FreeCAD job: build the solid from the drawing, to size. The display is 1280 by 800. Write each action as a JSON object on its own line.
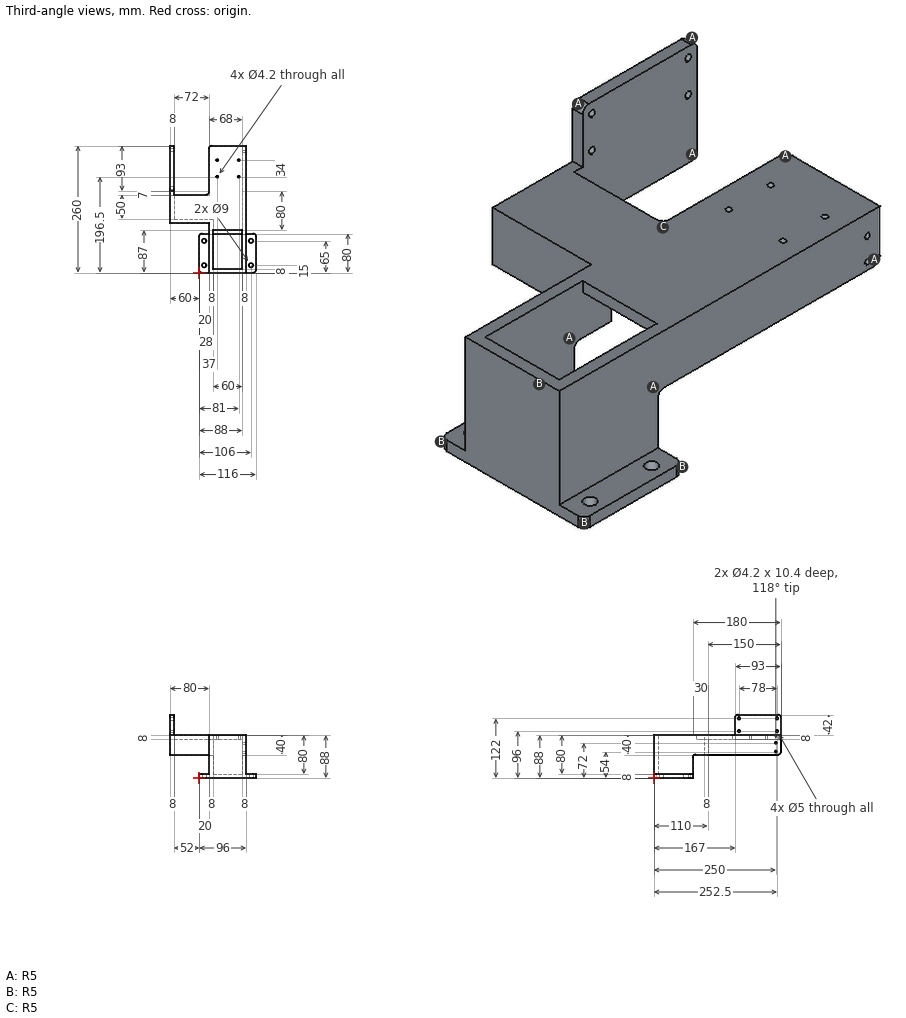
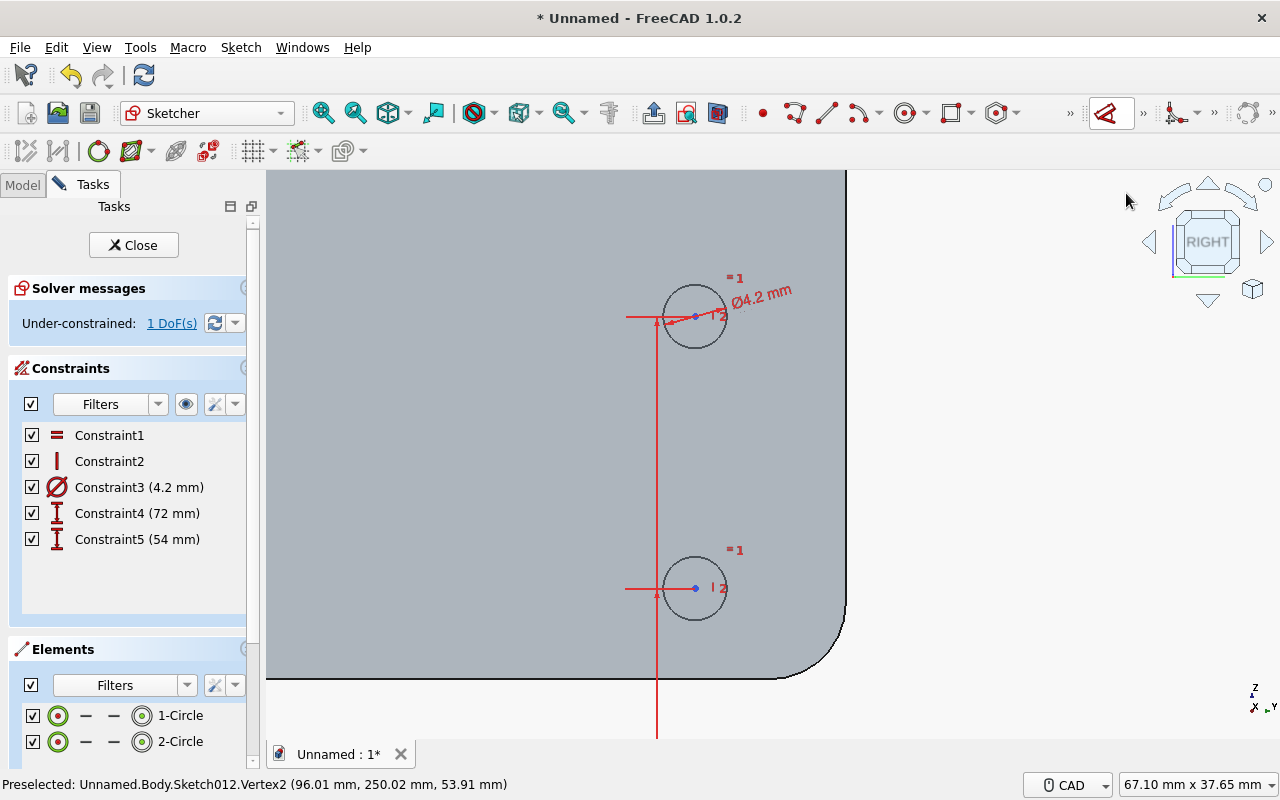
{"action": "left_click", "coordinate": [695, 317]}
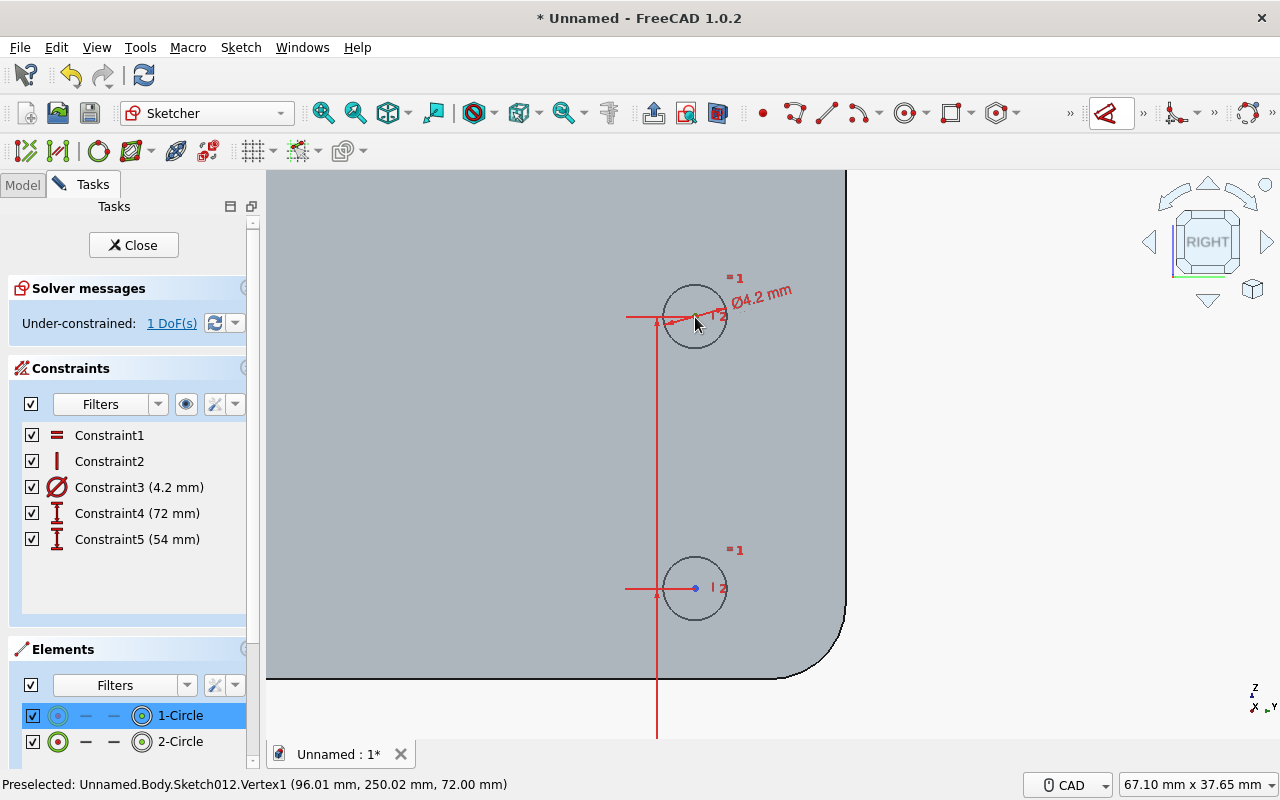
{"action": "left_click", "coordinate": [1128, 114]}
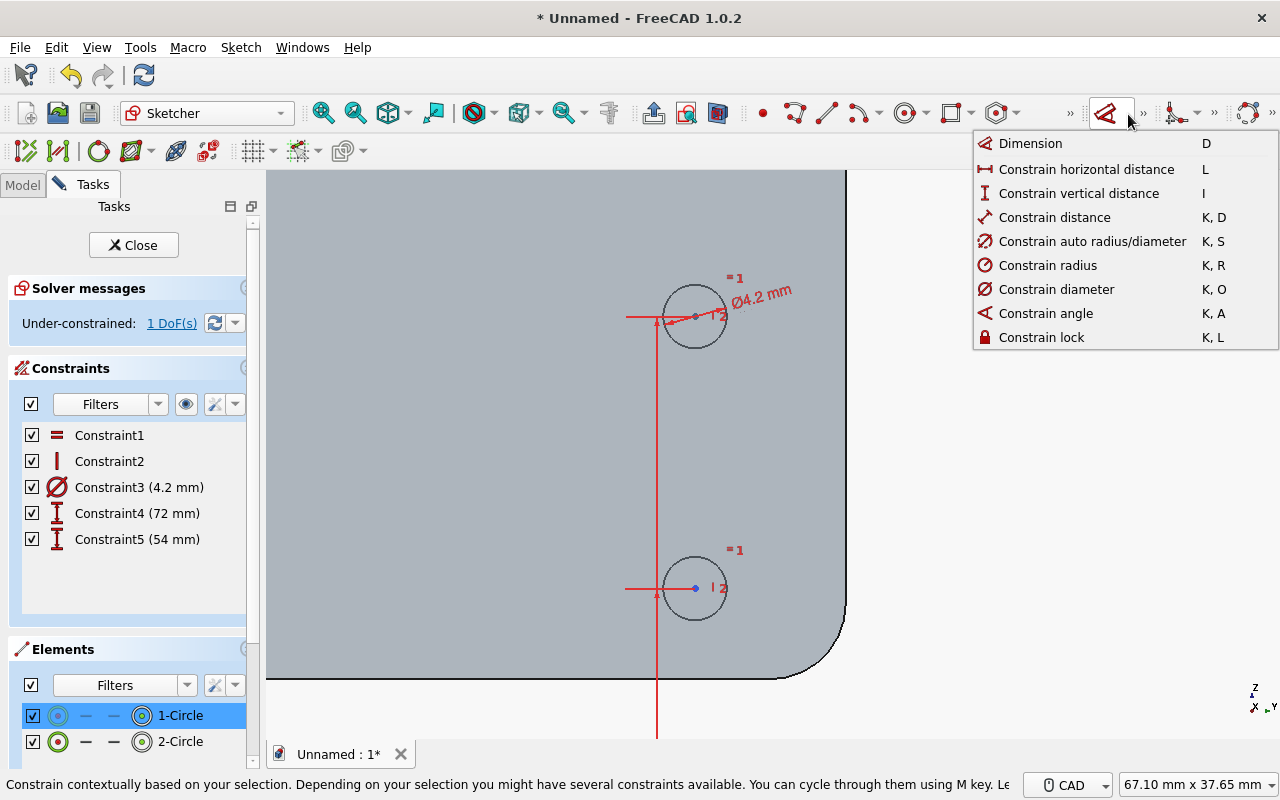
{"action": "left_click", "coordinate": [1126, 169]}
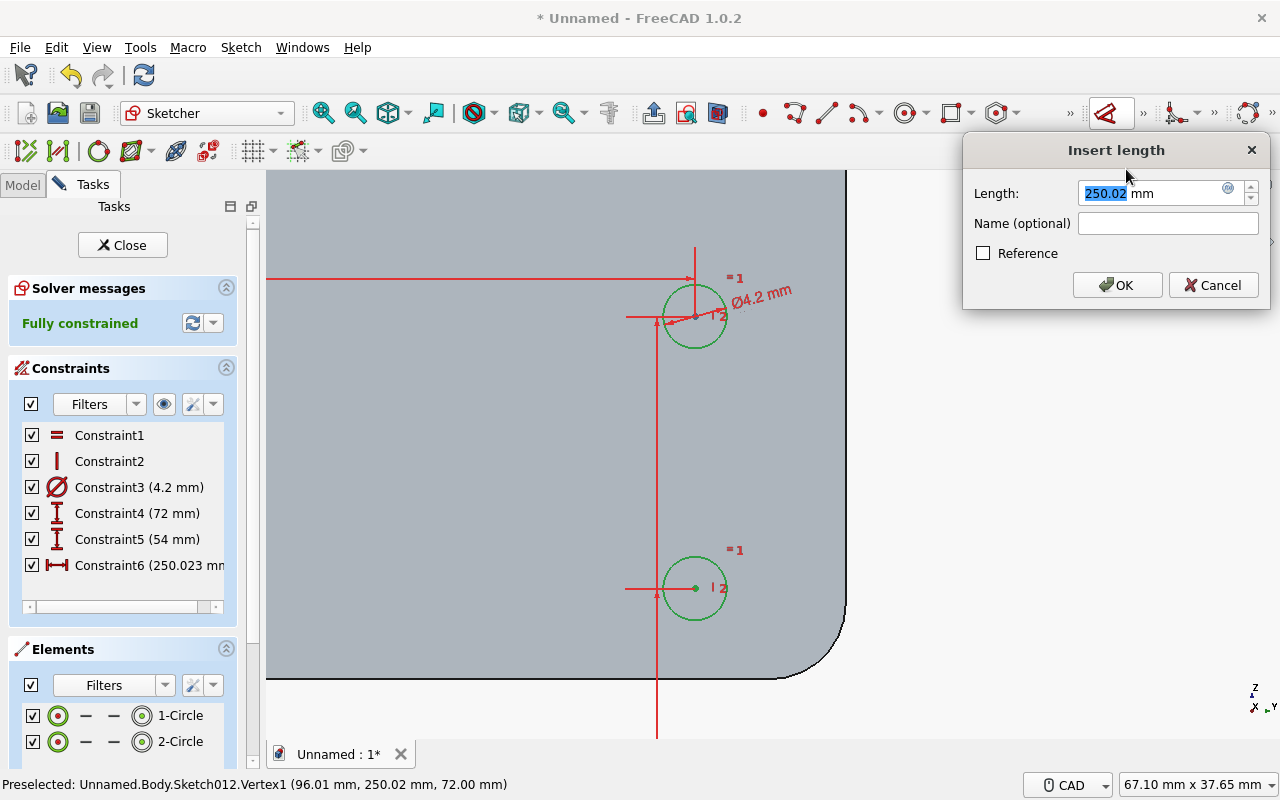
{"action": "type", "text": "250"}
{"action": "key", "text": "Return"}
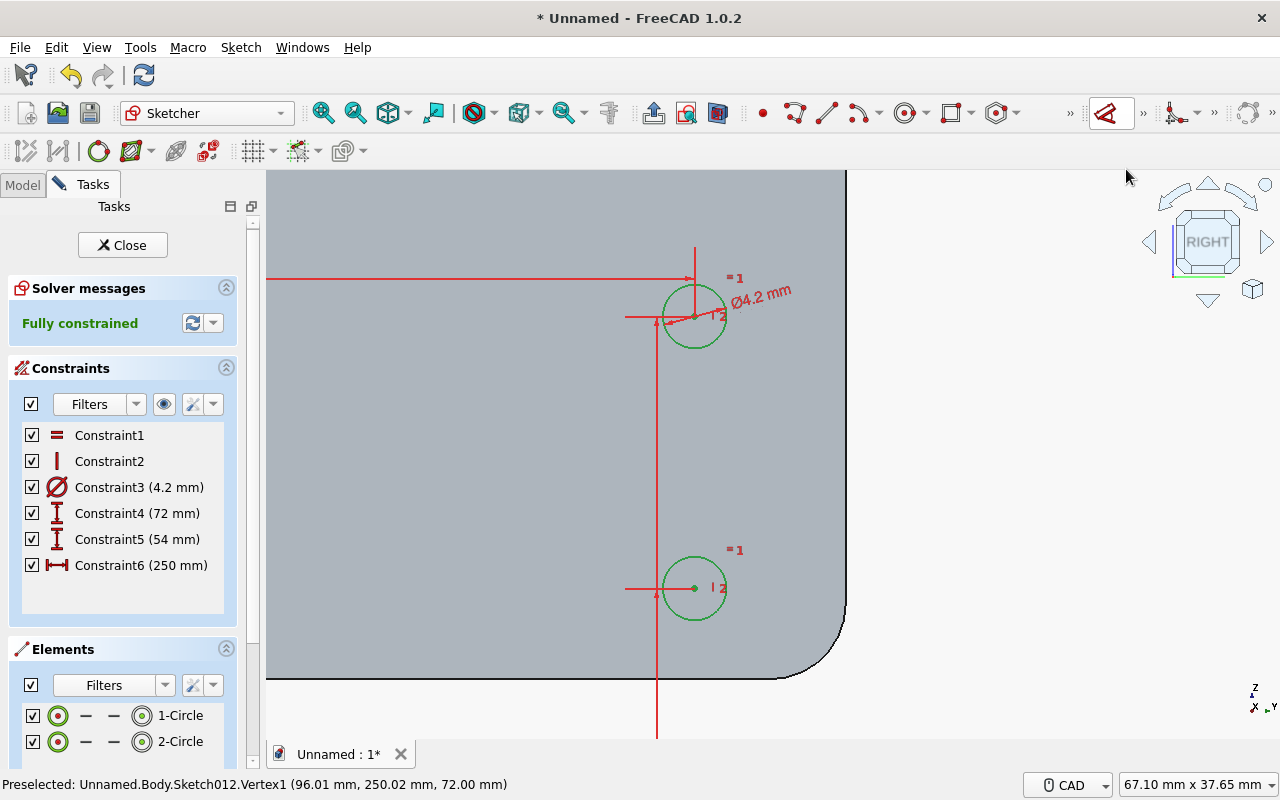
{"action": "left_click", "coordinate": [123, 245]}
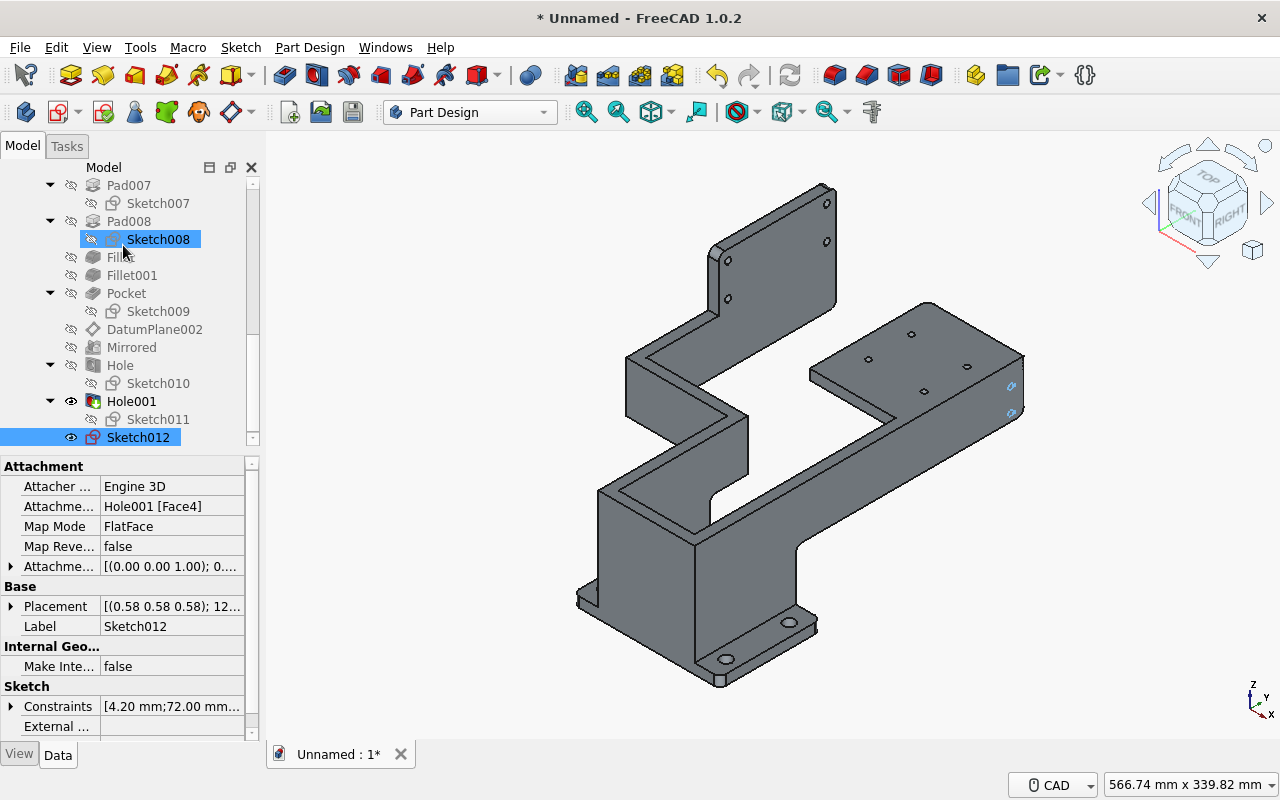
{"action": "left_click", "coordinate": [318, 76]}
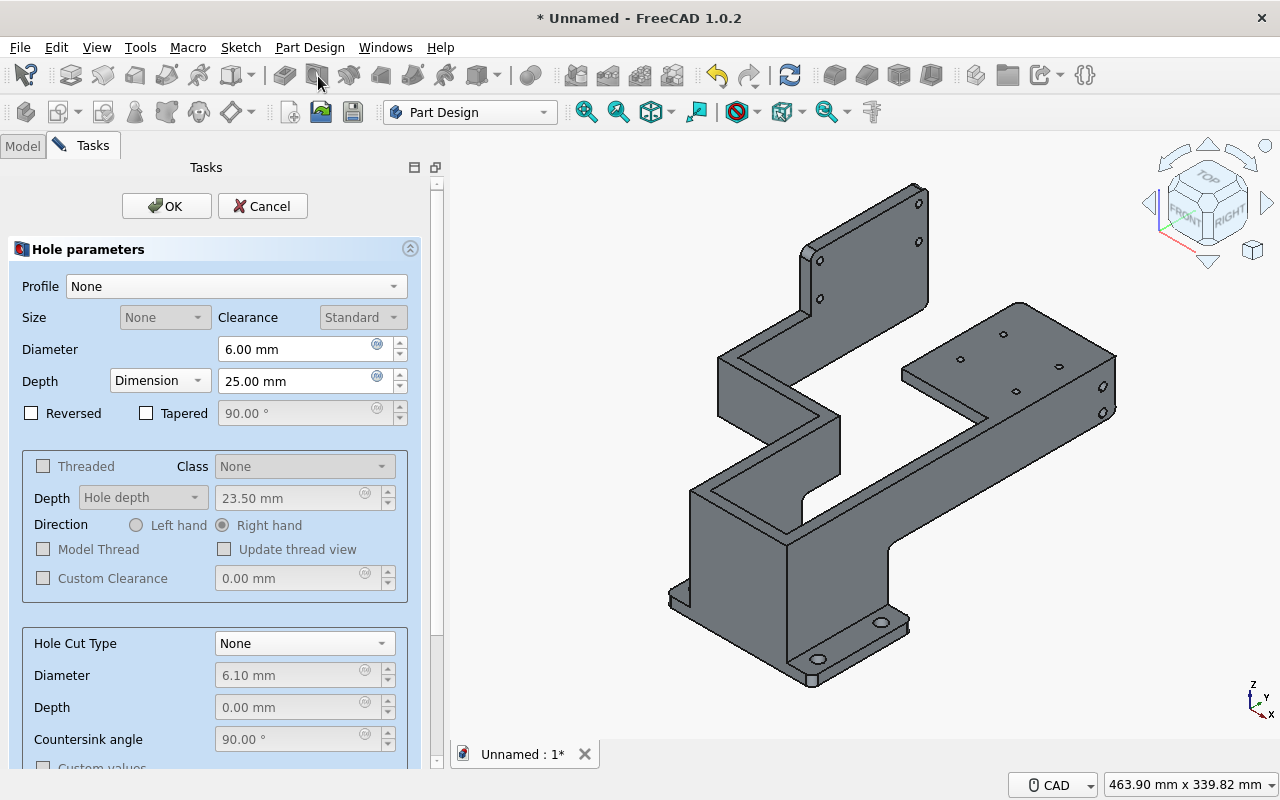
{"action": "triple_click", "coordinate": [305, 349]}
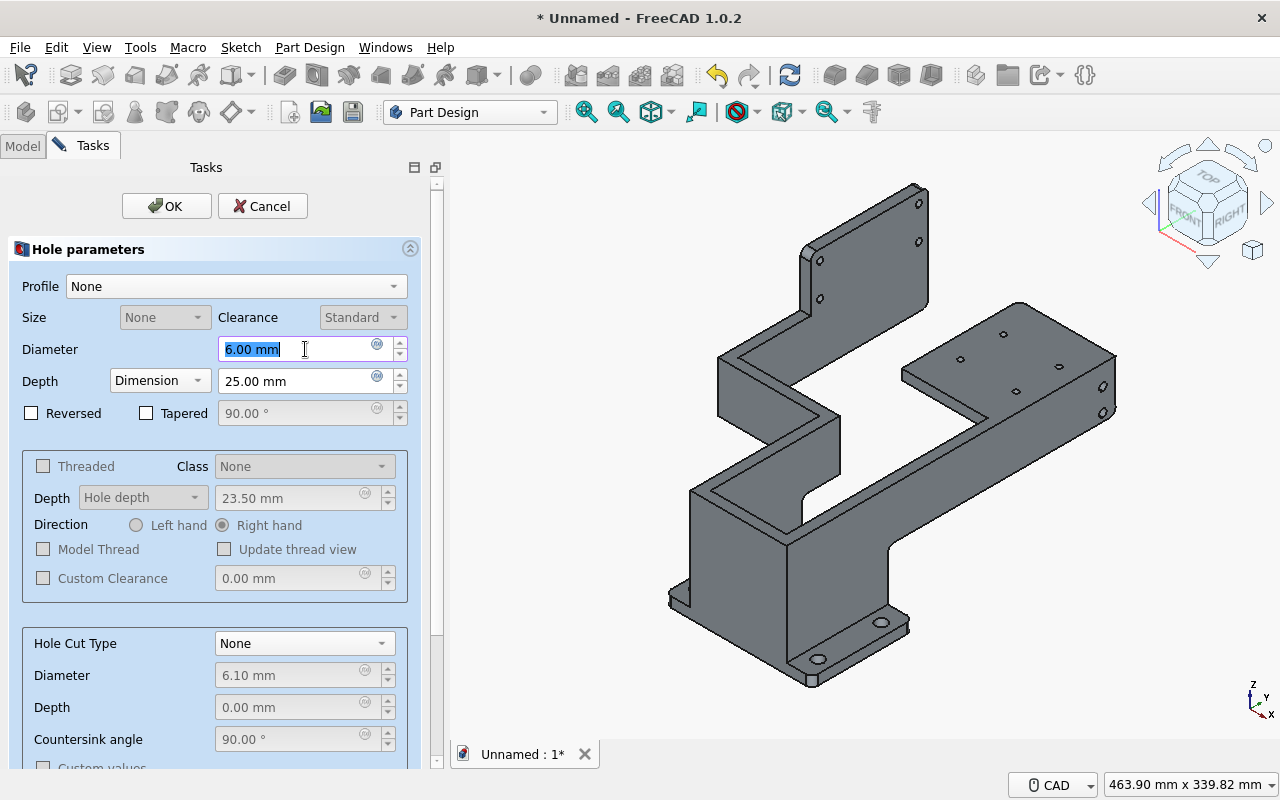
{"action": "type", "text": "4.2"}
{"action": "key", "text": "Tab"}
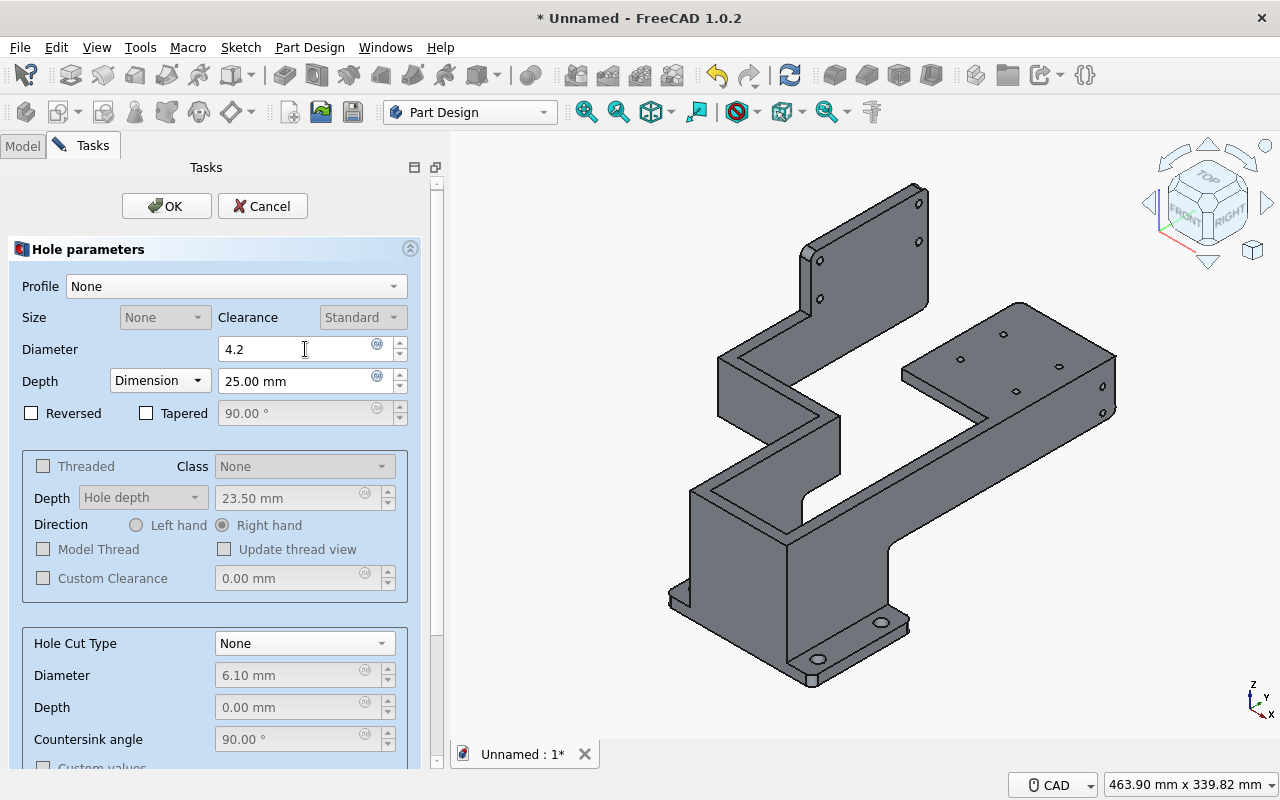
{"action": "triple_click", "coordinate": [305, 381]}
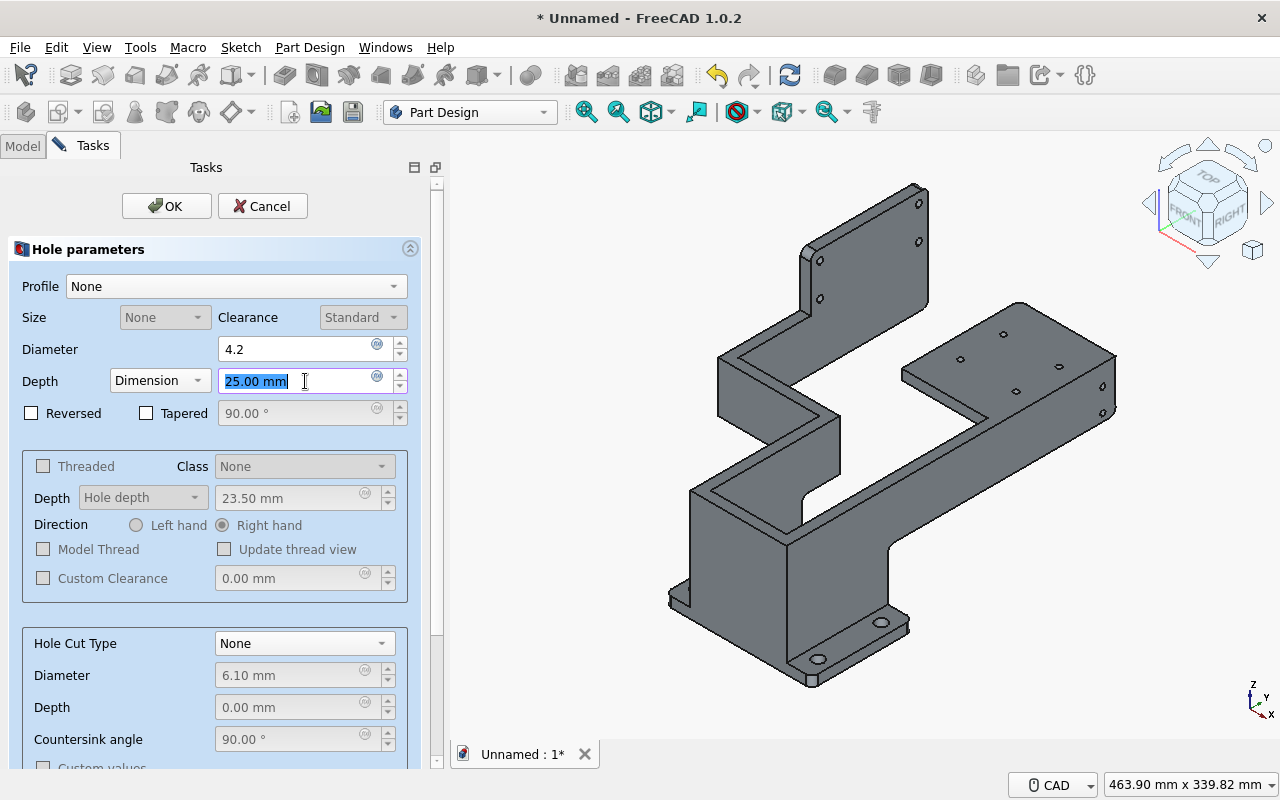
{"action": "type", "text": "10.4"}
{"action": "key", "text": "Tab"}